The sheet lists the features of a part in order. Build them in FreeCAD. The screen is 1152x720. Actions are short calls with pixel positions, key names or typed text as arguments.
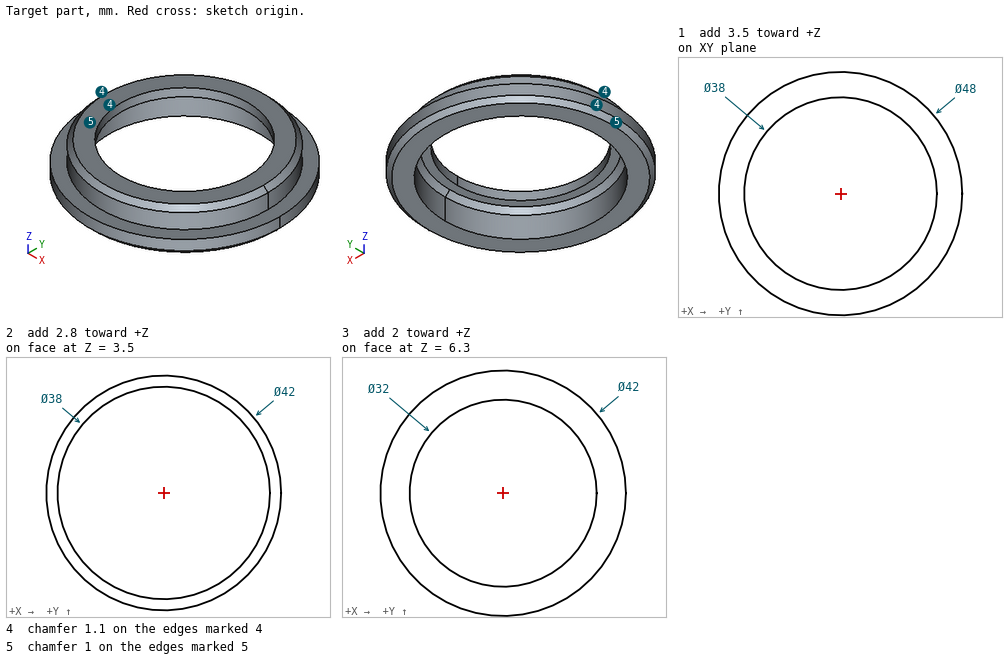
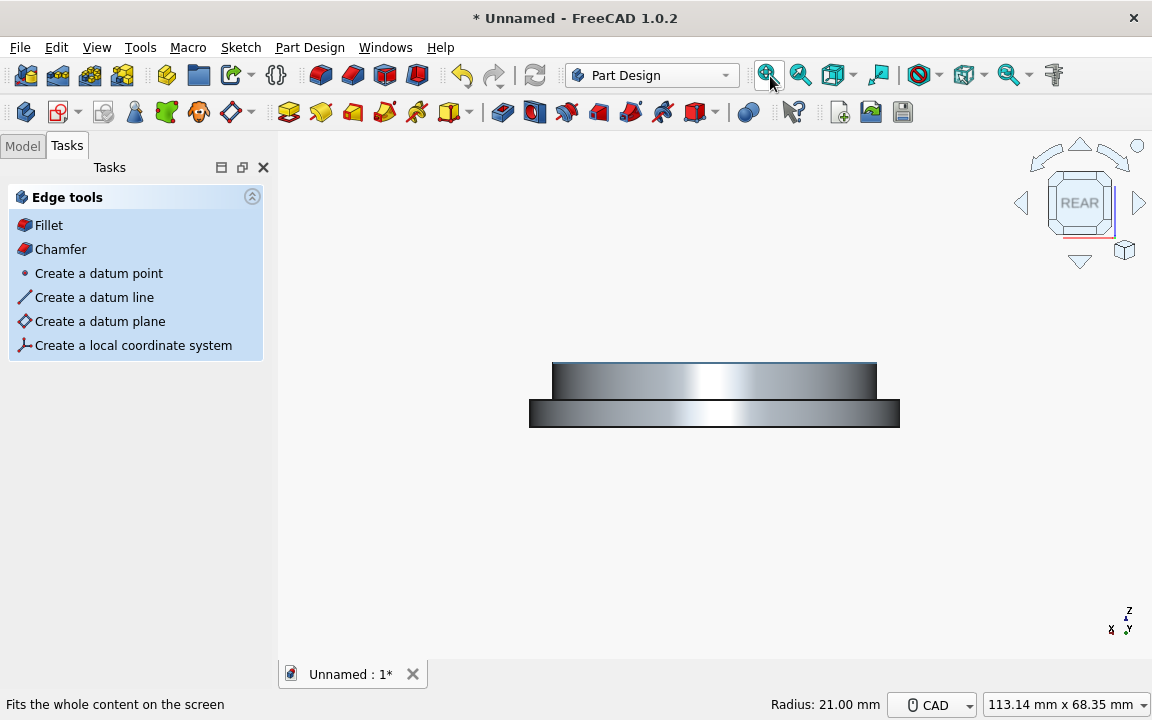
click(770, 76)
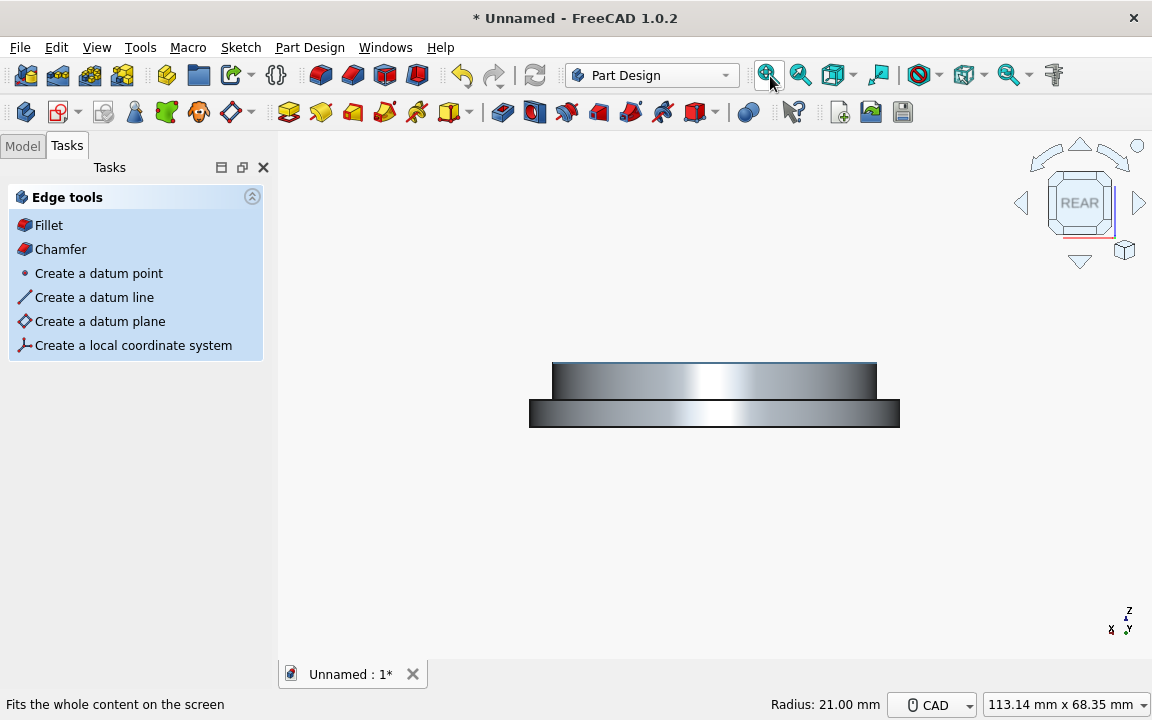
key(6)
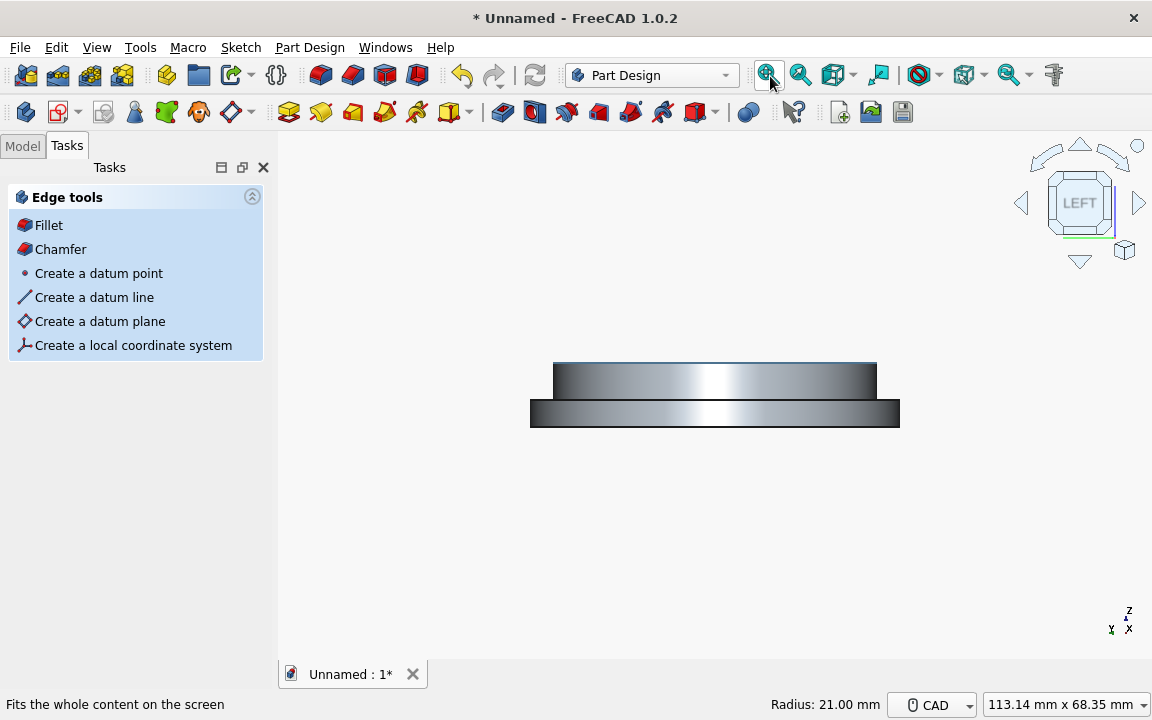
click(770, 76)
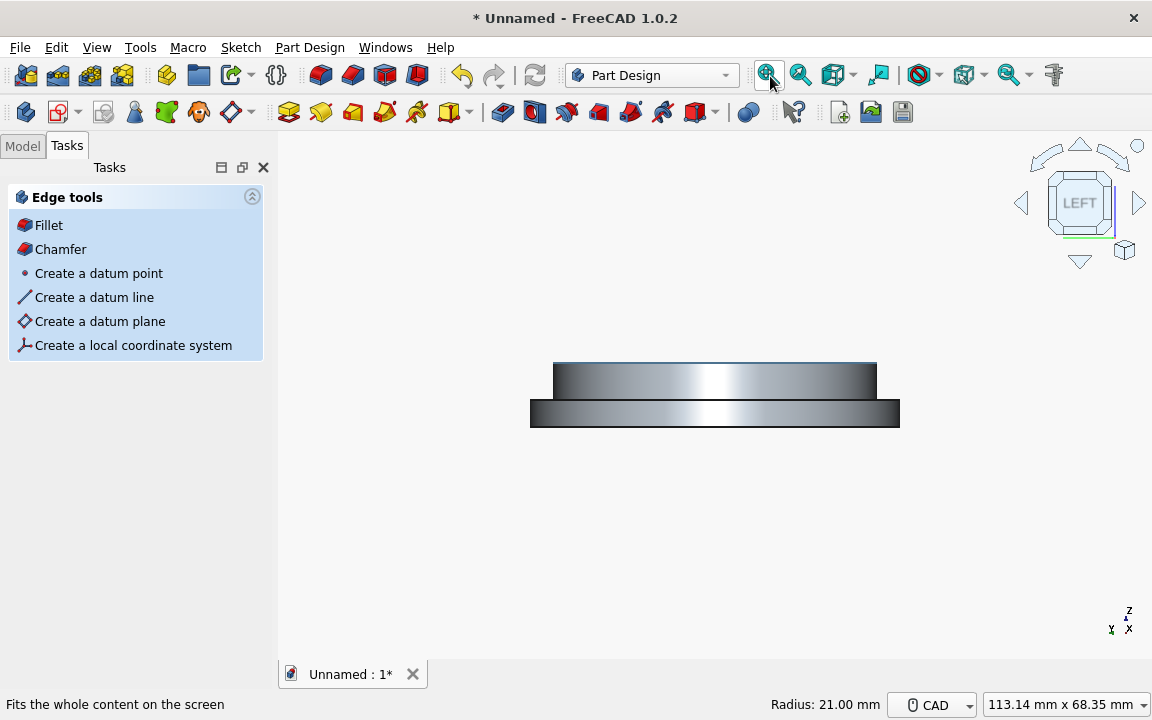
key(v)
key(3)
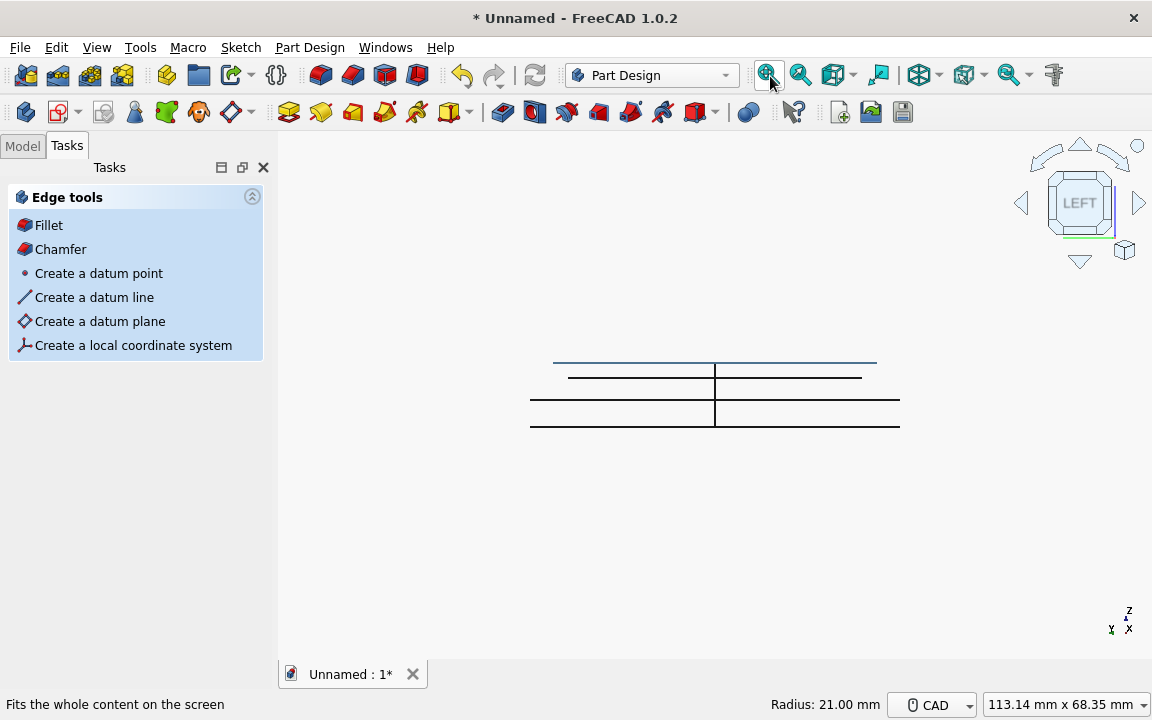
key(0)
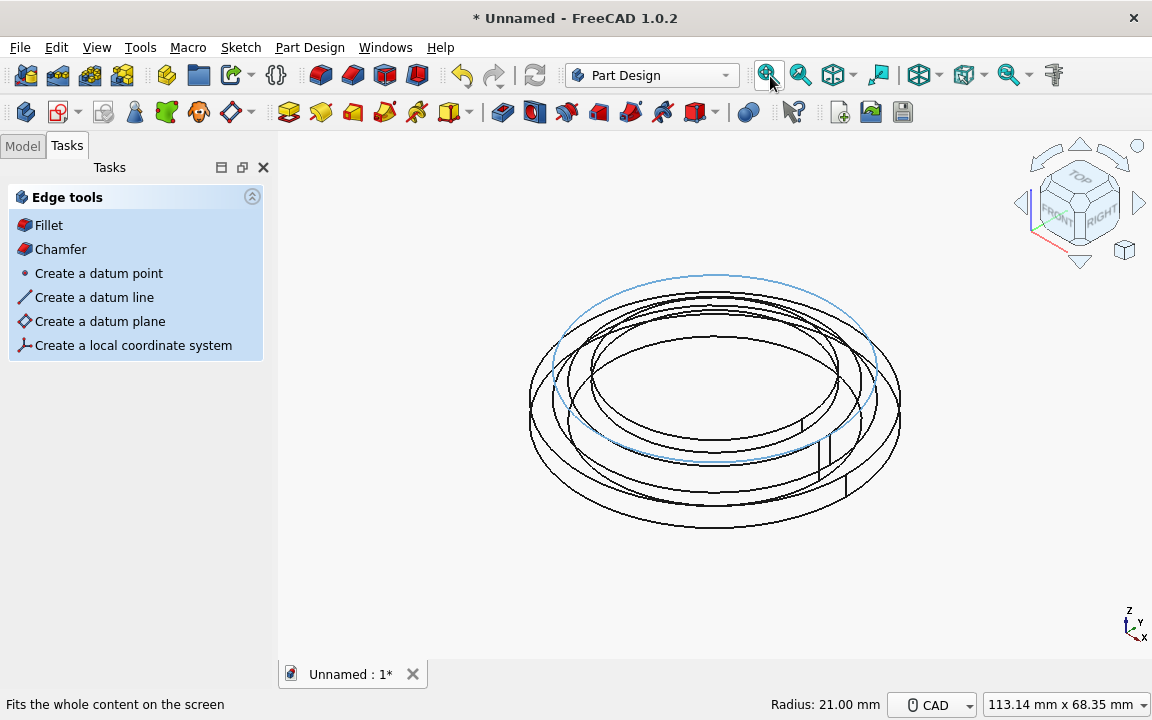
click(611, 320, ctrl)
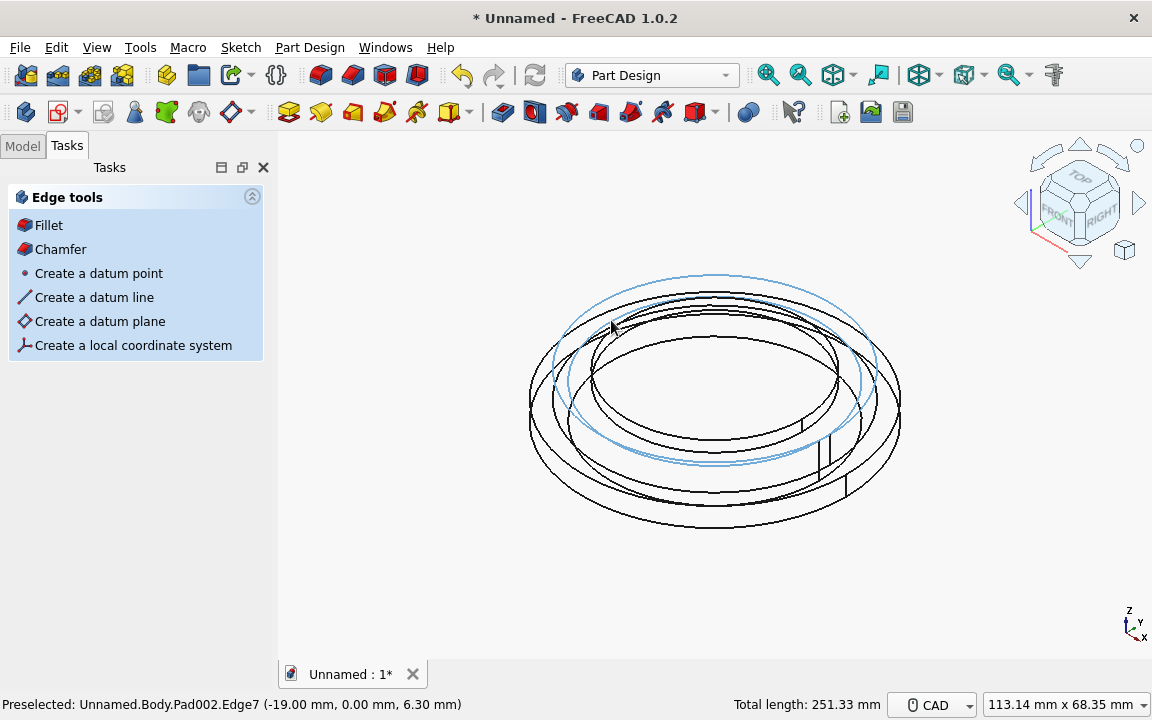
key(v)
key(1)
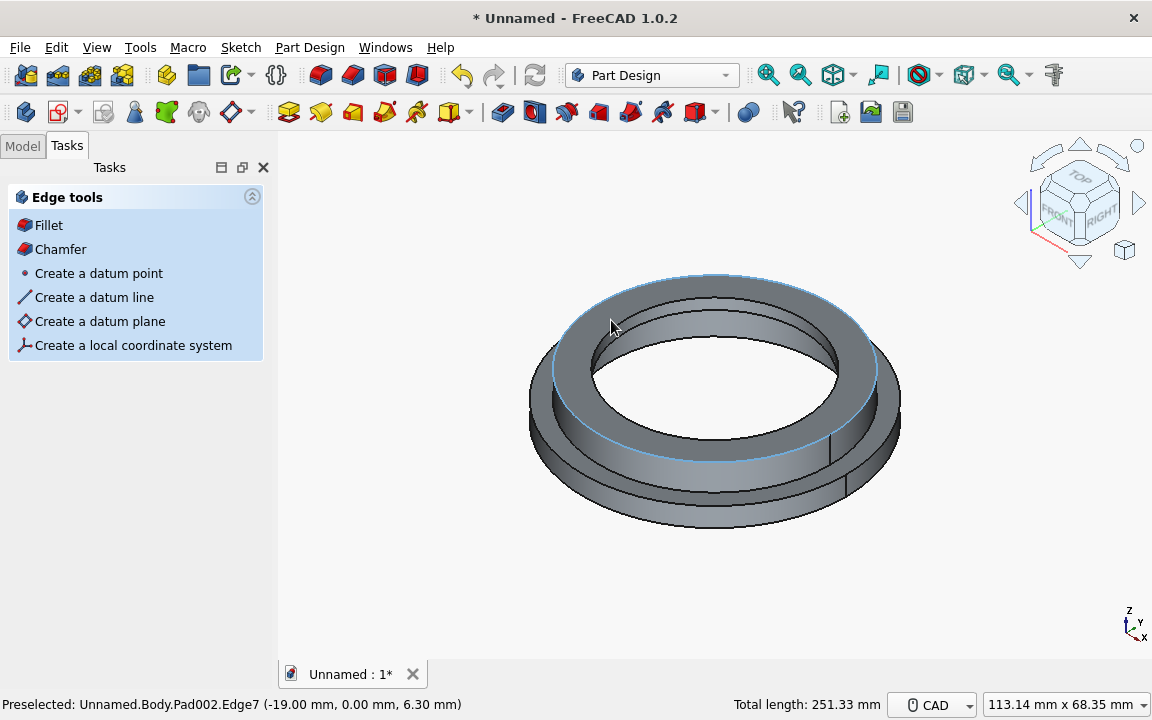
click(354, 76)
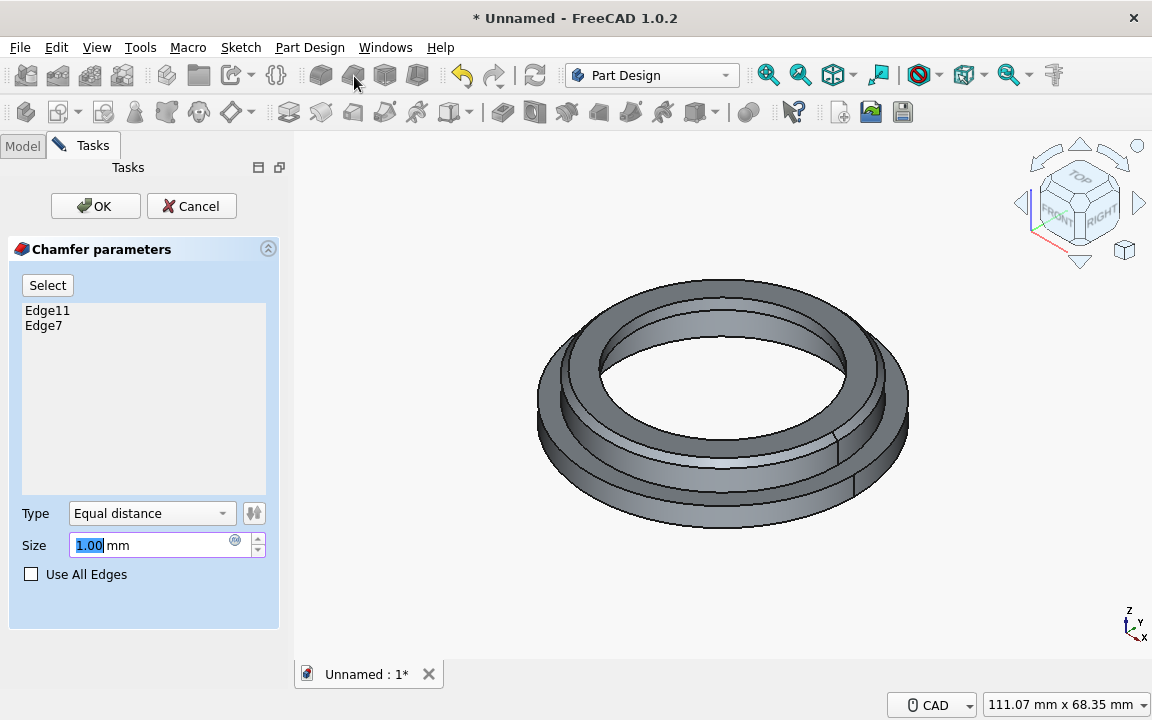
text(1.1)
key(Tab)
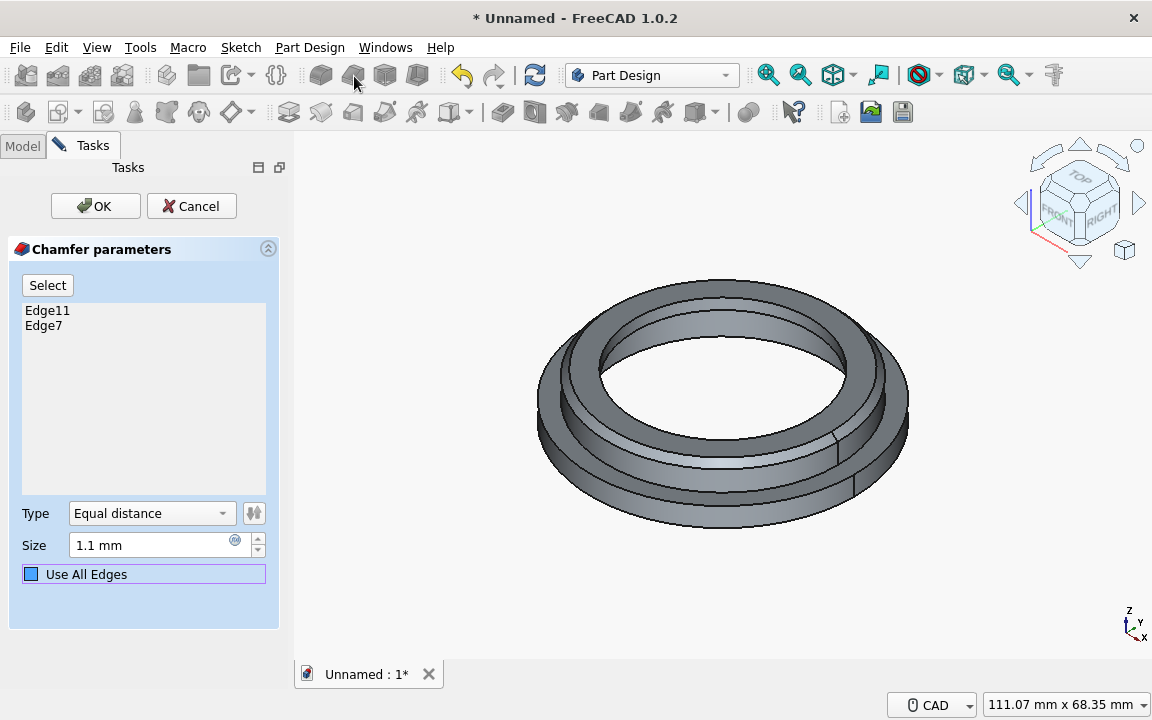
click(96, 206)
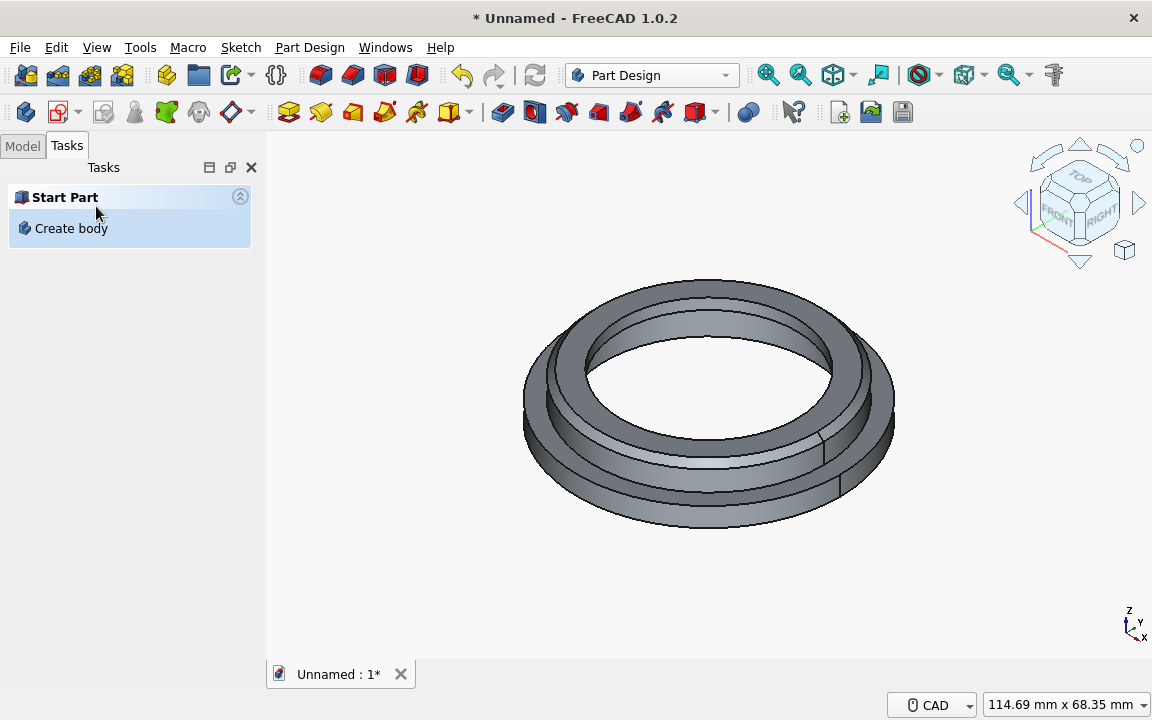
key(2)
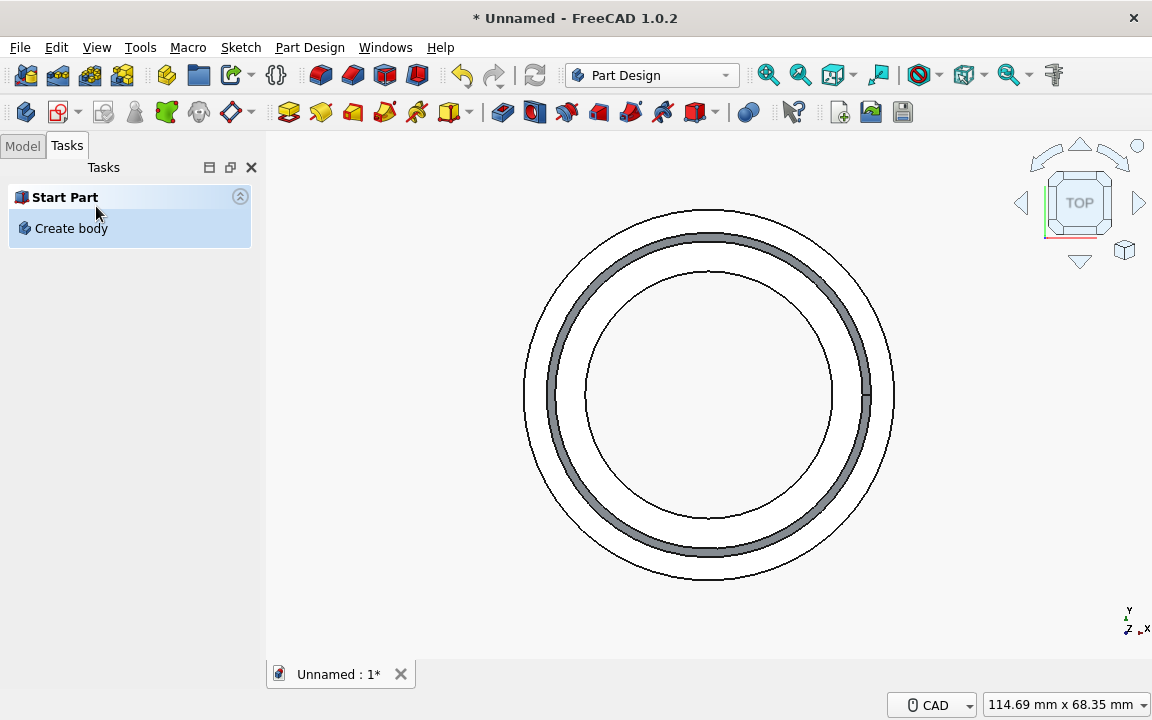
key(0)